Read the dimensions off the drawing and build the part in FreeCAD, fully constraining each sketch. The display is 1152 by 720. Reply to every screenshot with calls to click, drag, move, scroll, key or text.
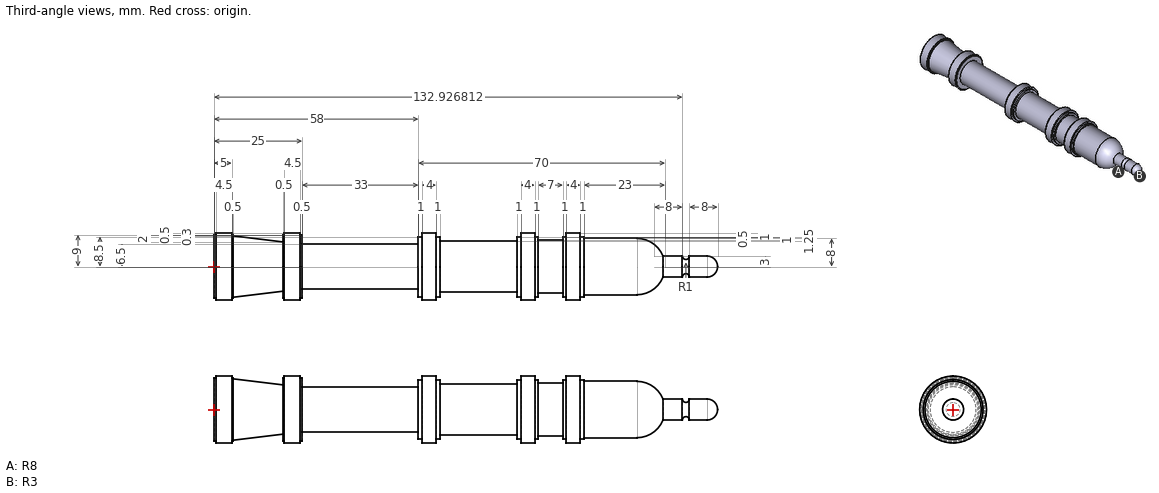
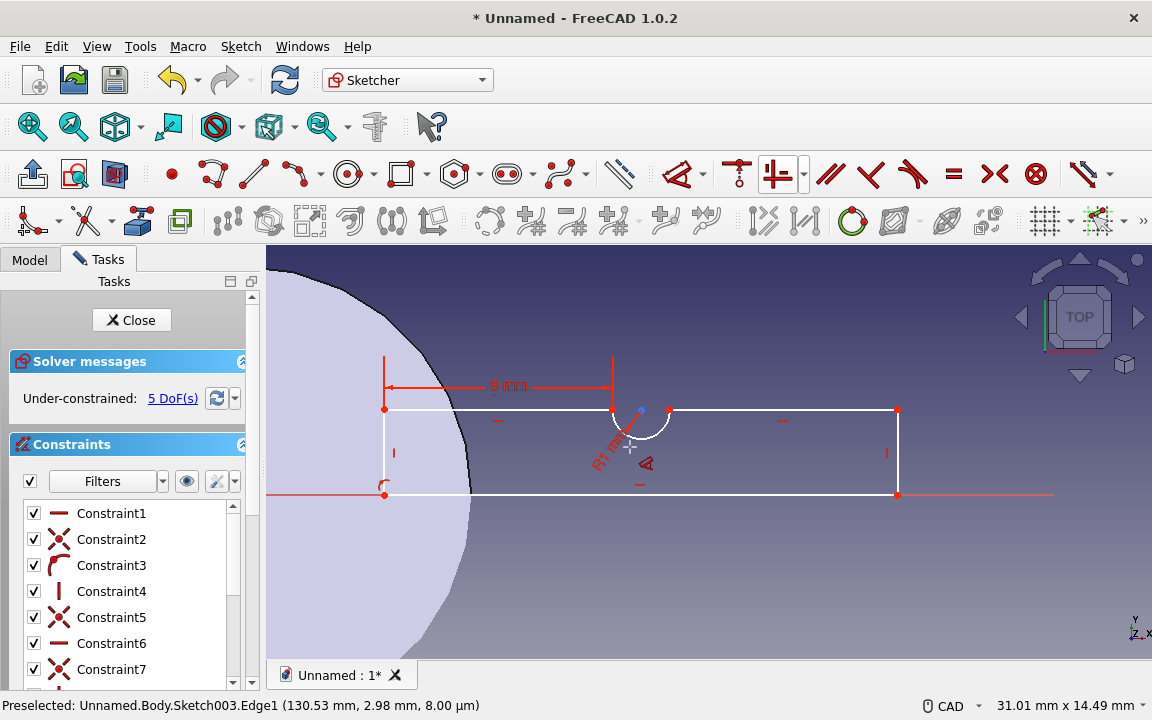
click(384, 436)
click(350, 453)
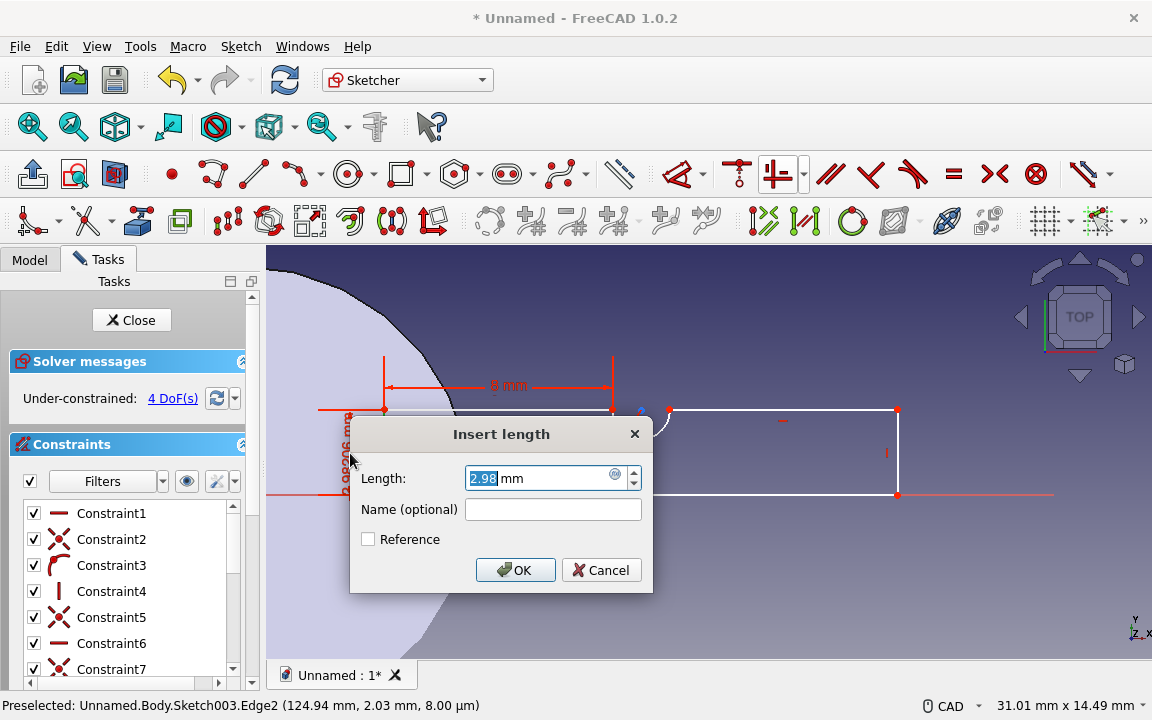
text(3)
key(Return)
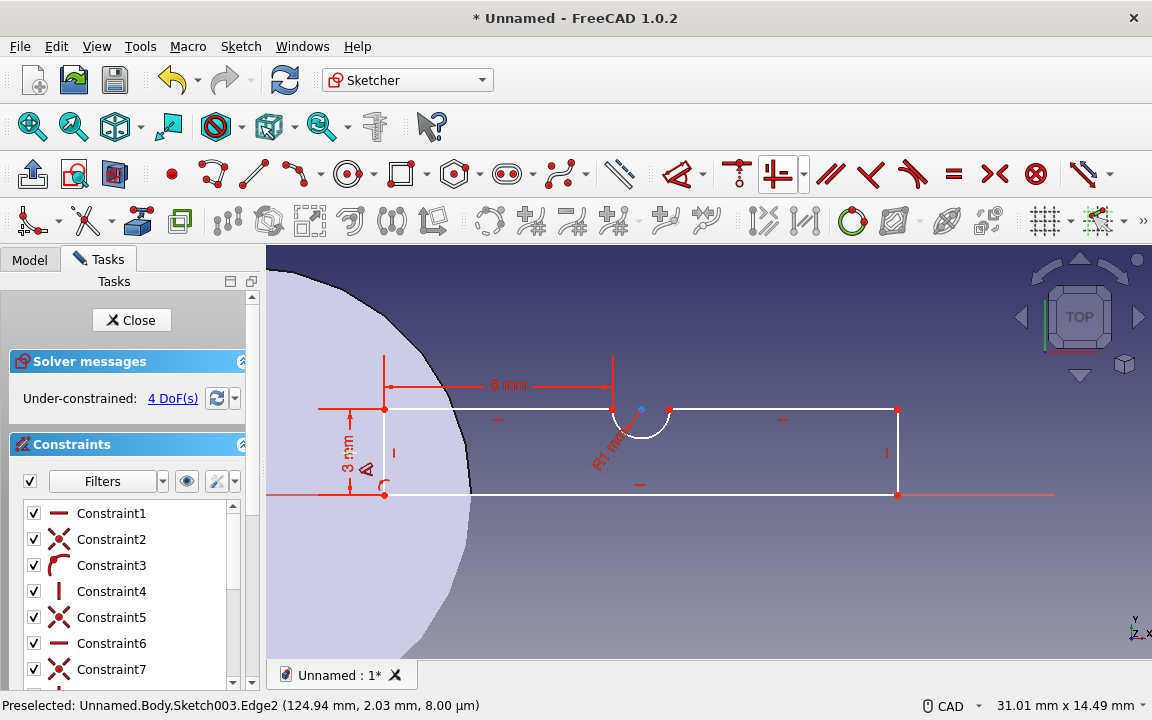
click(898, 469)
click(932, 452)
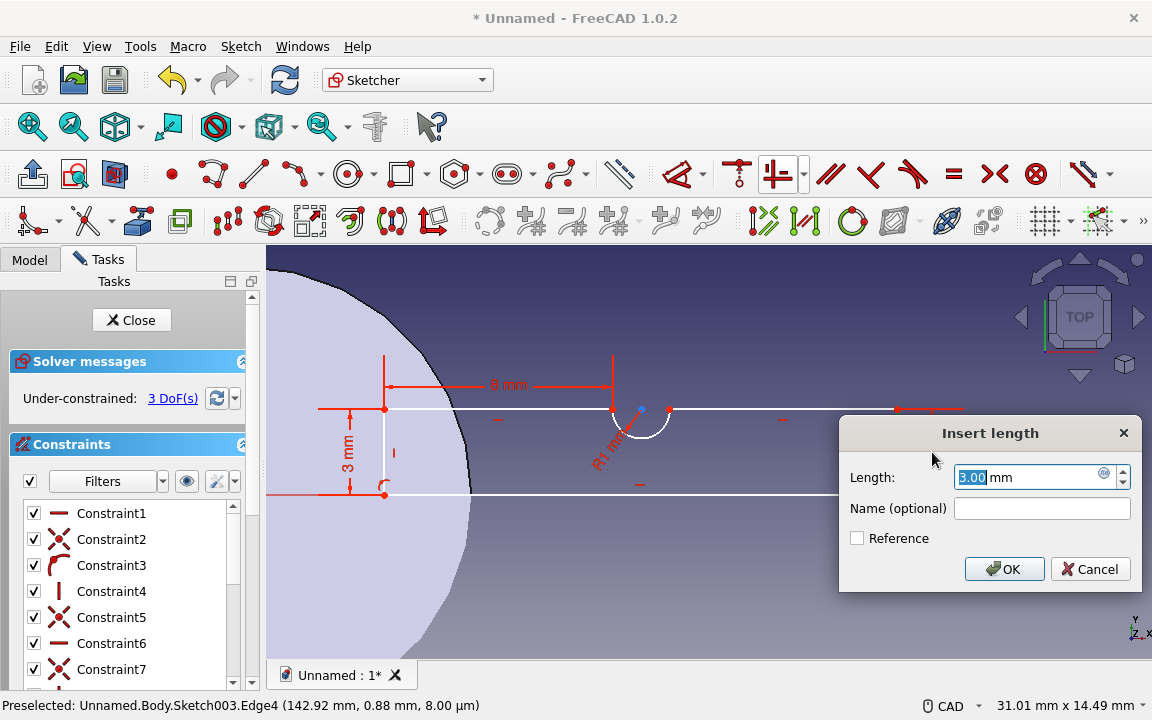
text(3)
key(Return)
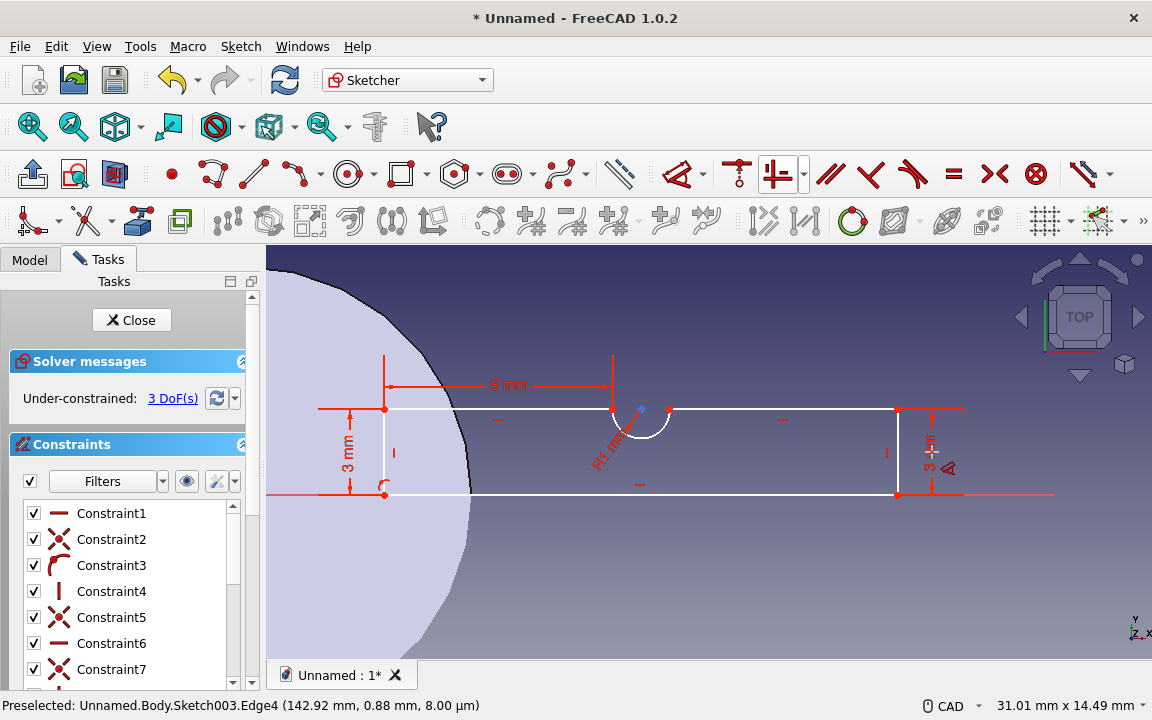
click(829, 409)
click(784, 375)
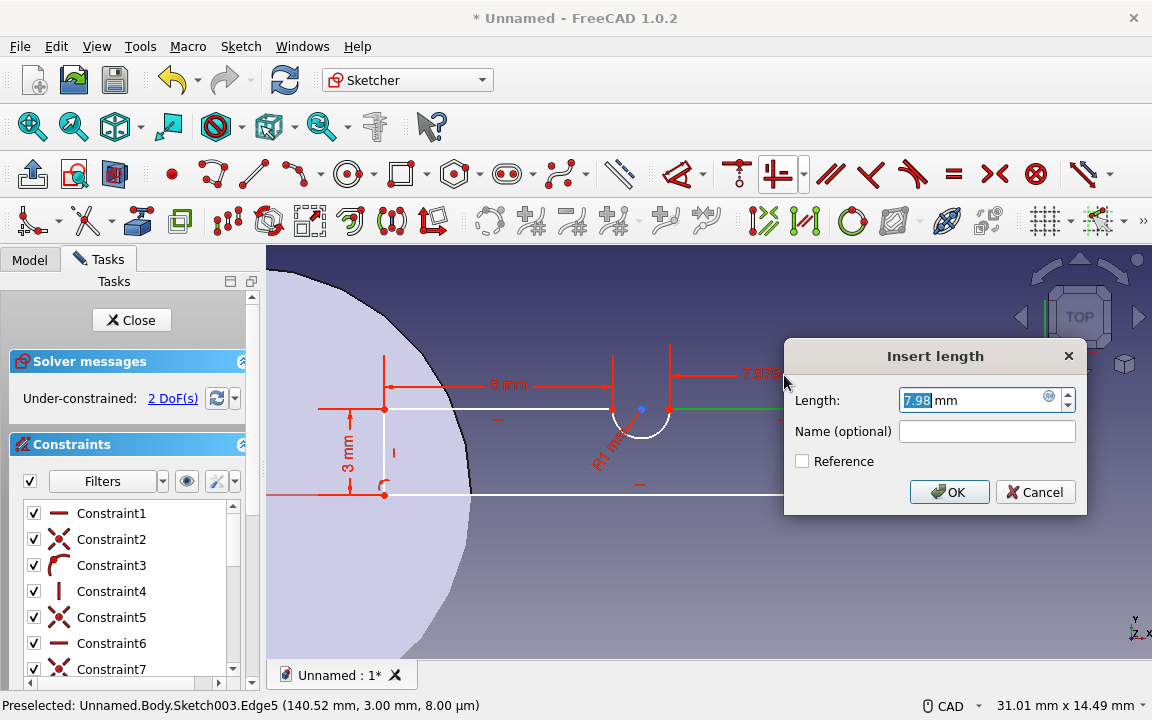
text(8)
key(Return)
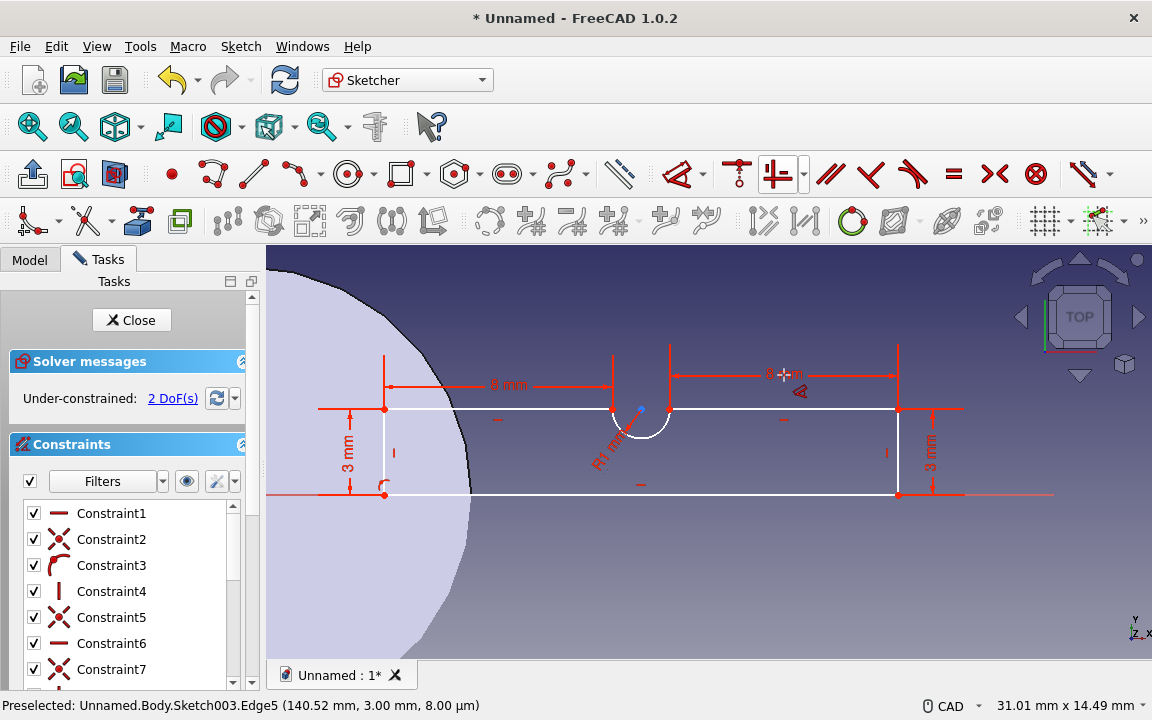
click(641, 410)
click(675, 472)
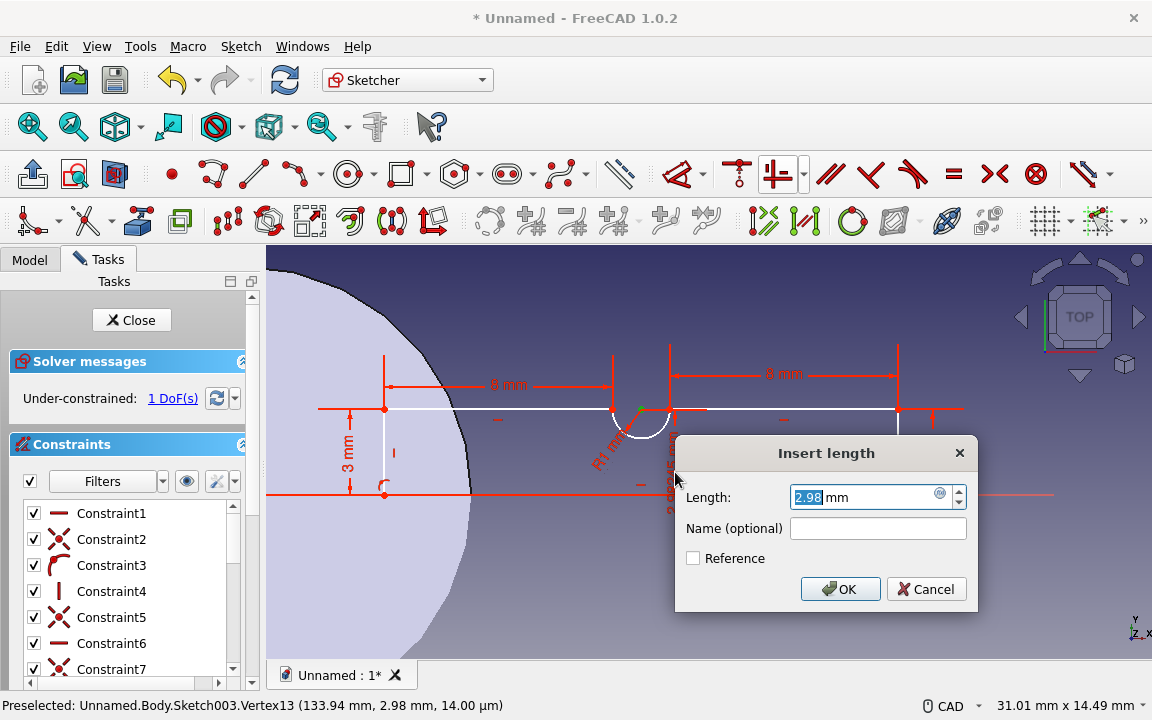
text(3)
key(Return)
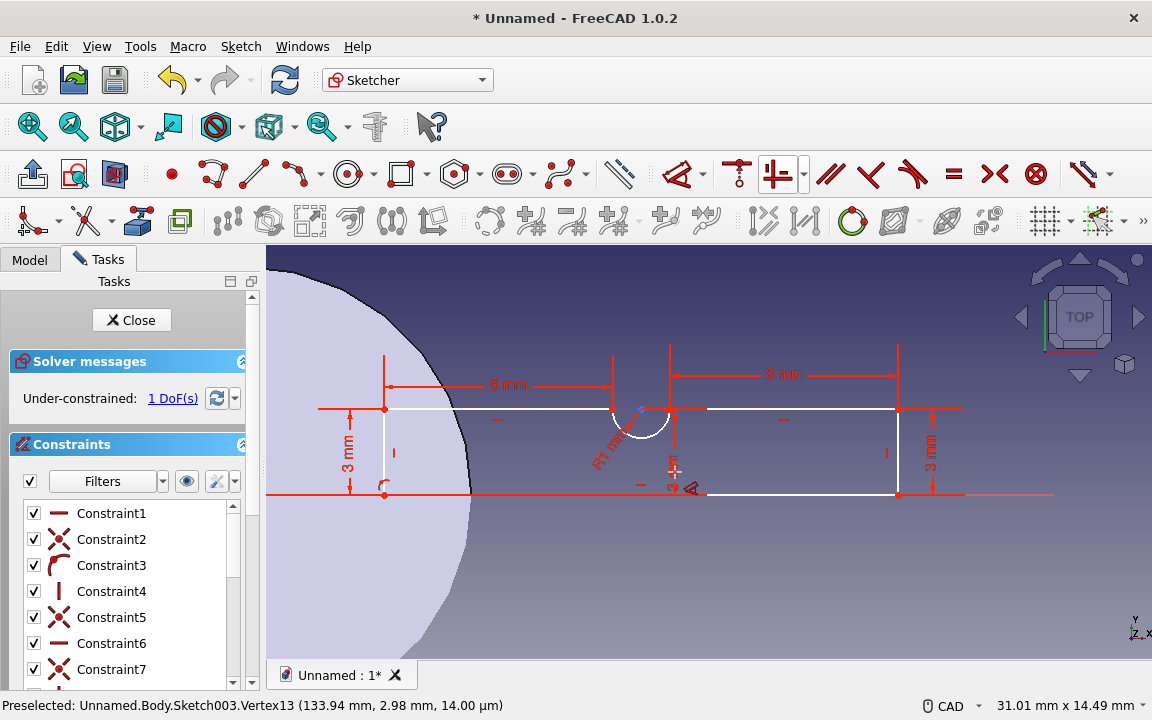
click(613, 409)
click(453, 529)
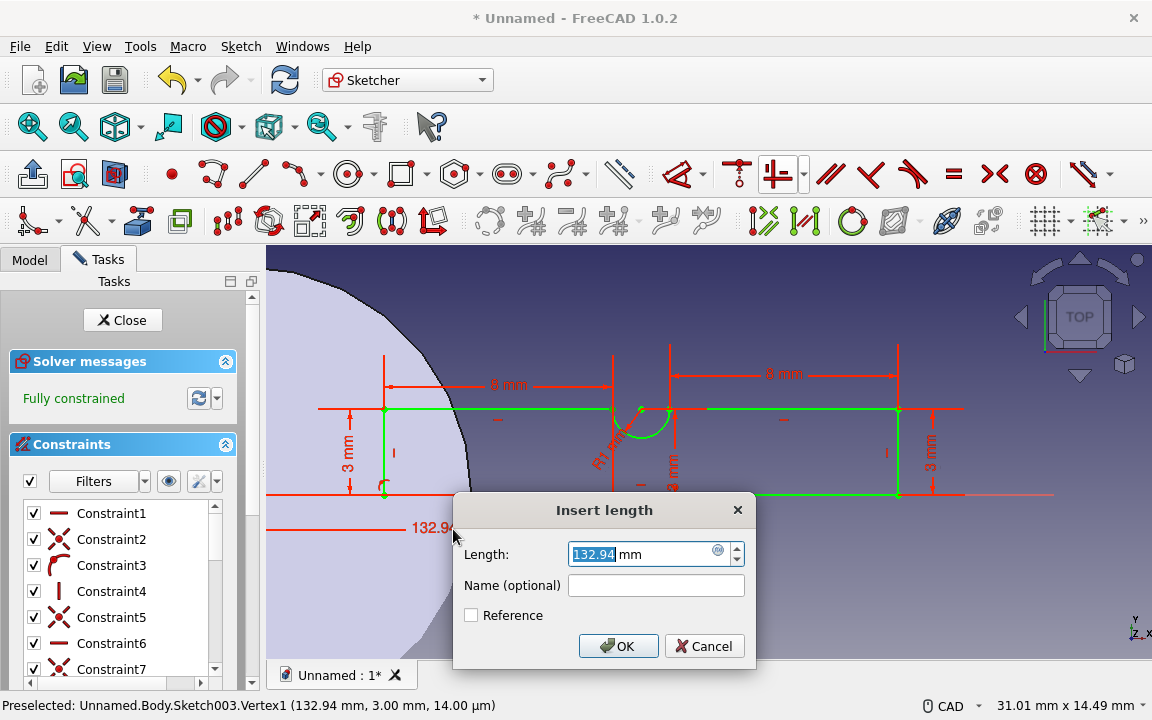
text(132.926812)
key(Return)
key(Escape)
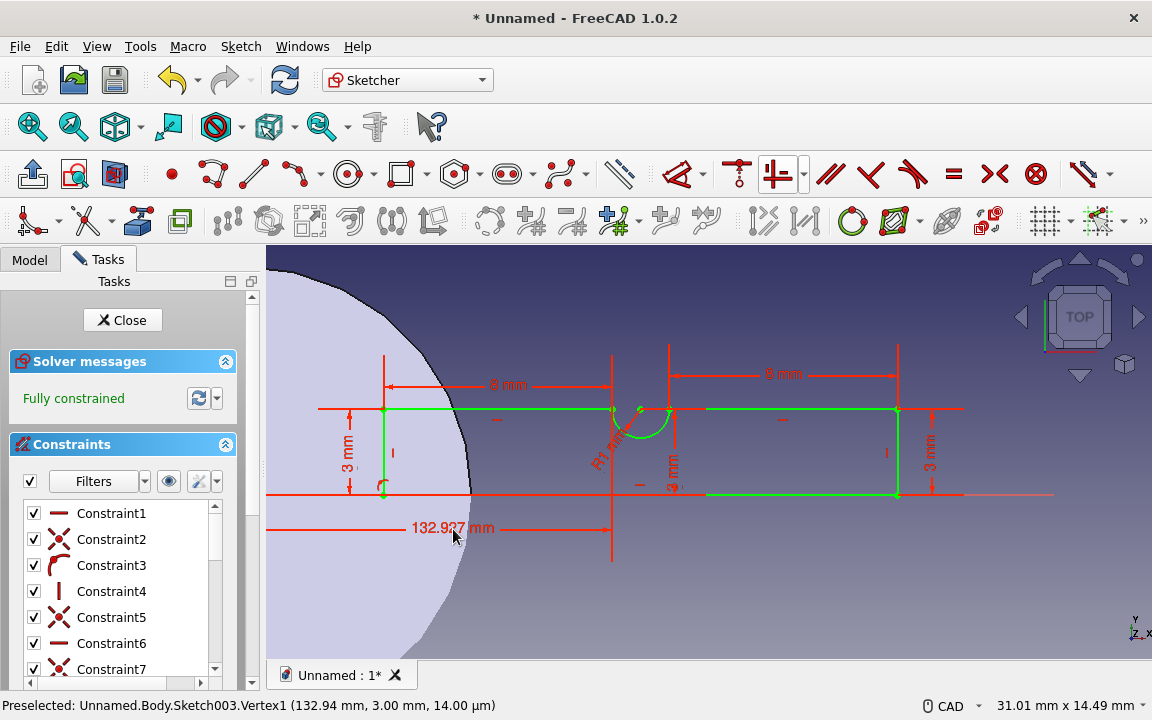
click(123, 320)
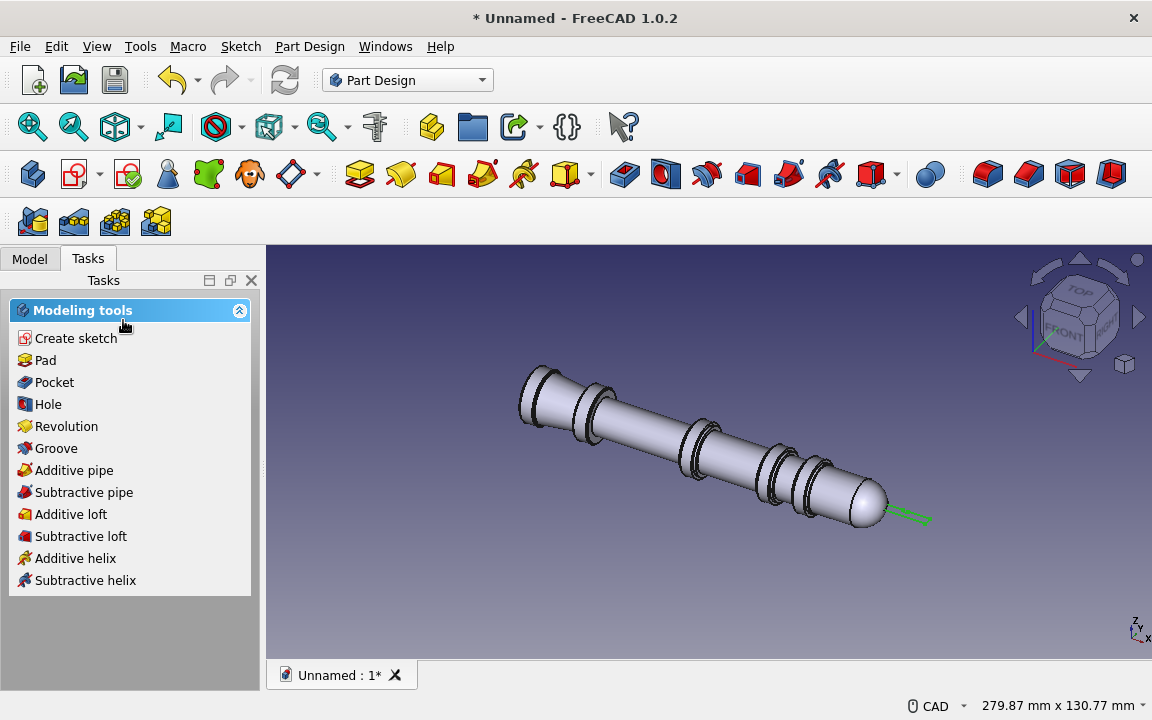
click(401, 174)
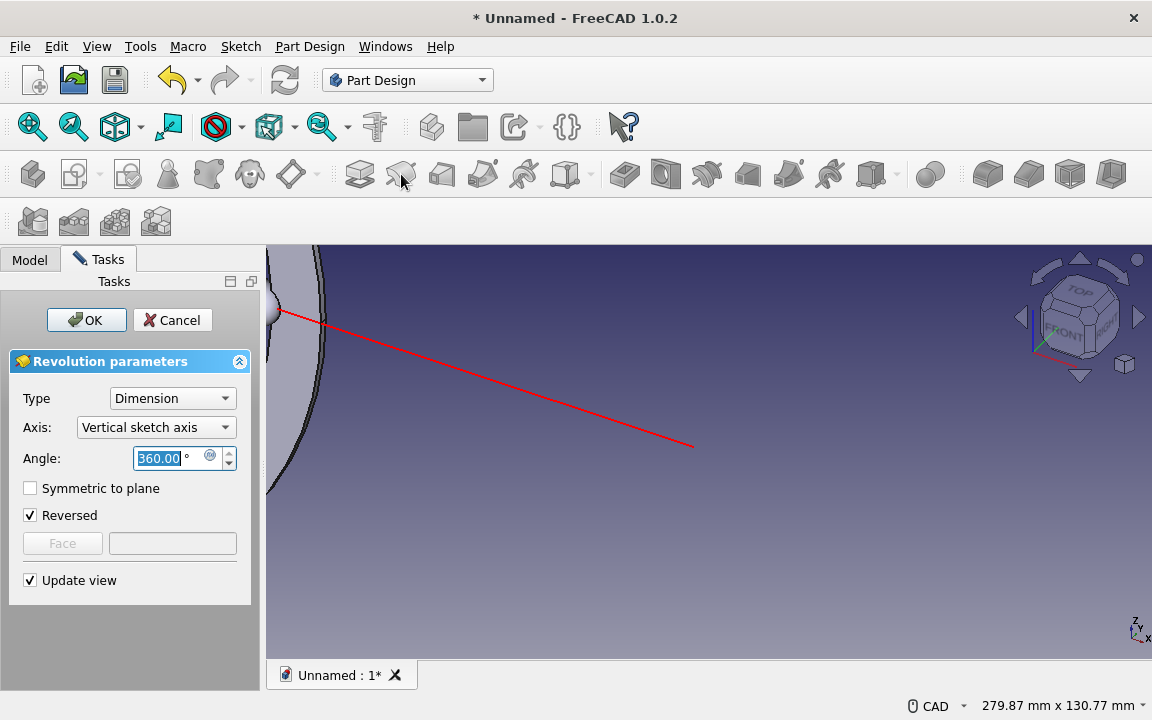
click(157, 428)